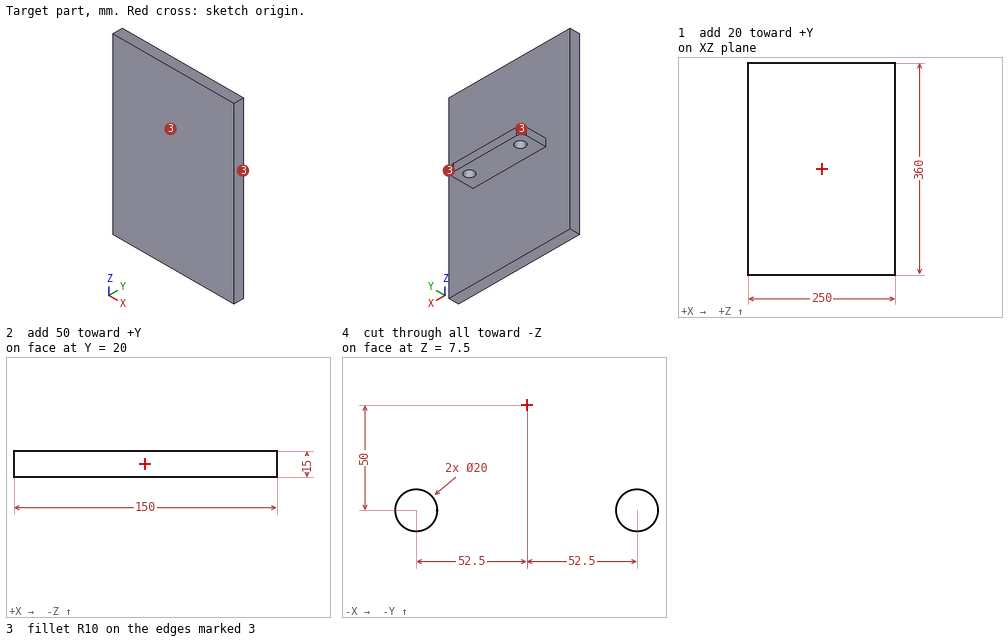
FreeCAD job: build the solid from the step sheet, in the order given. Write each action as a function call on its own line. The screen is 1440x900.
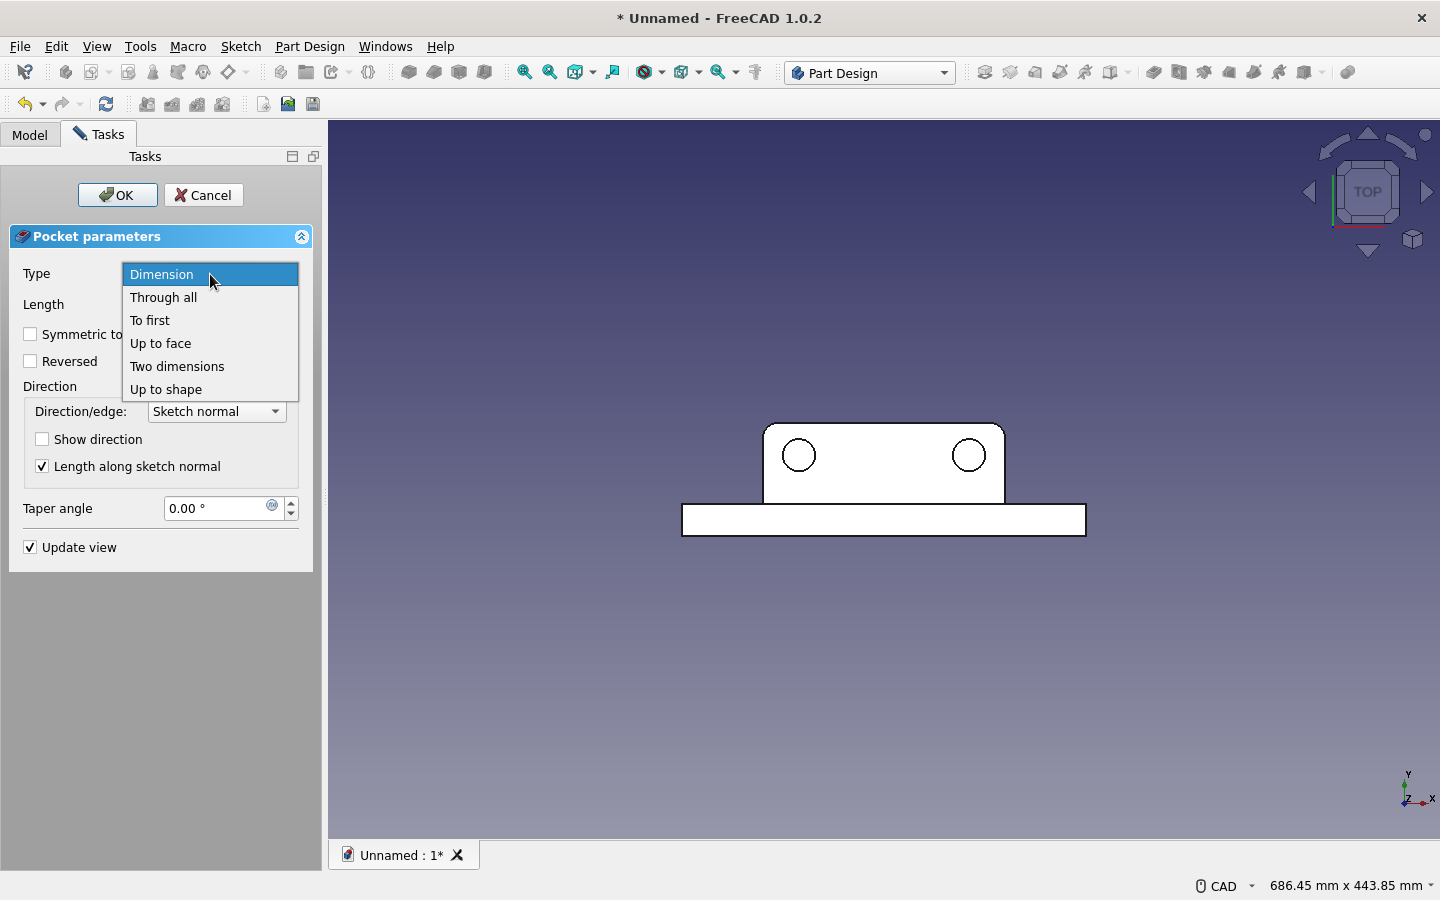
click(208, 298)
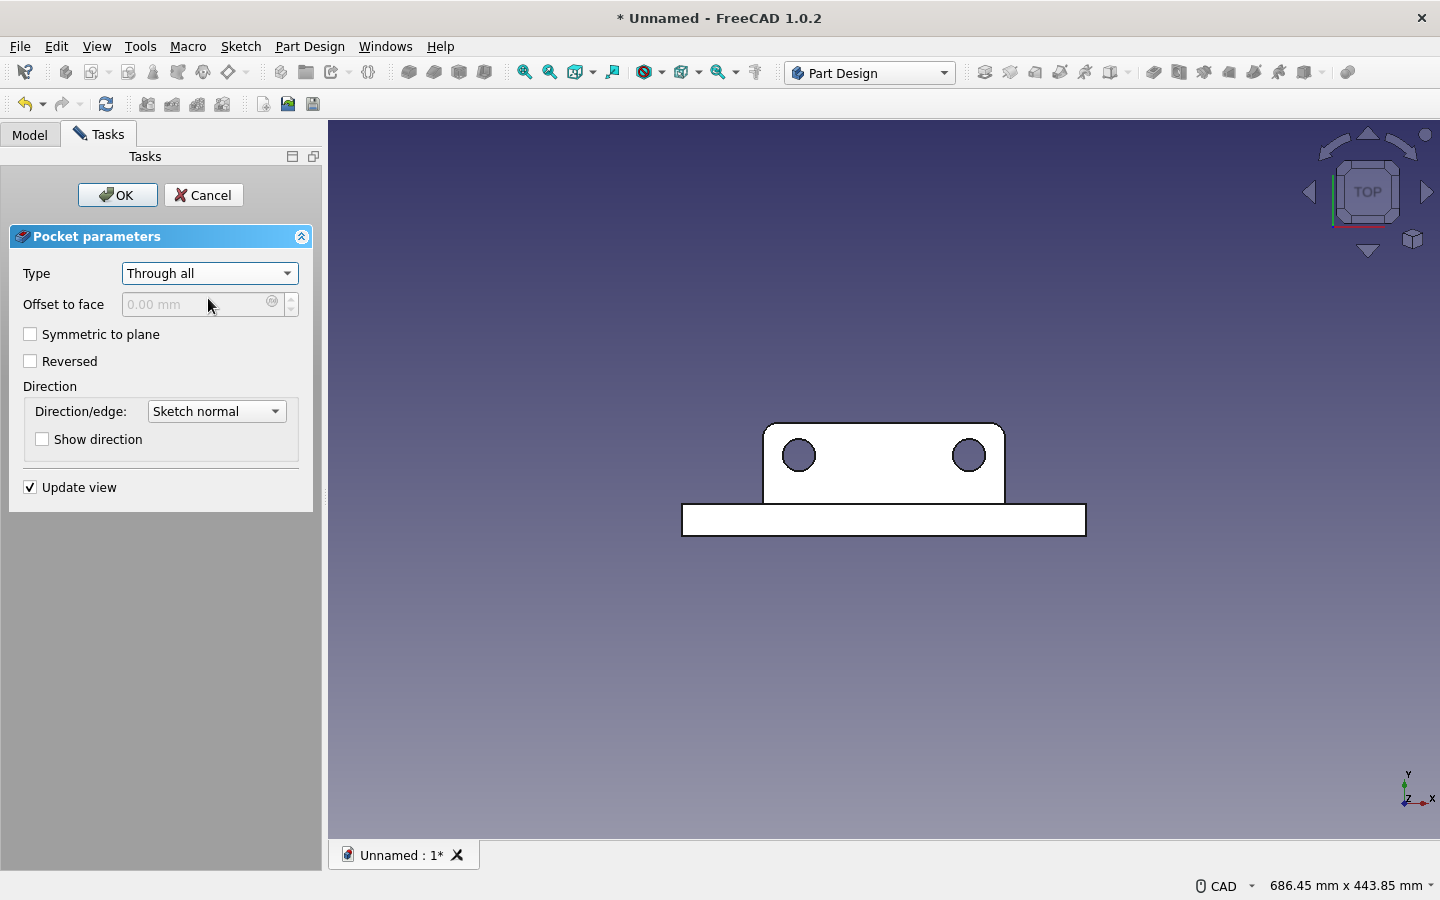
click(118, 195)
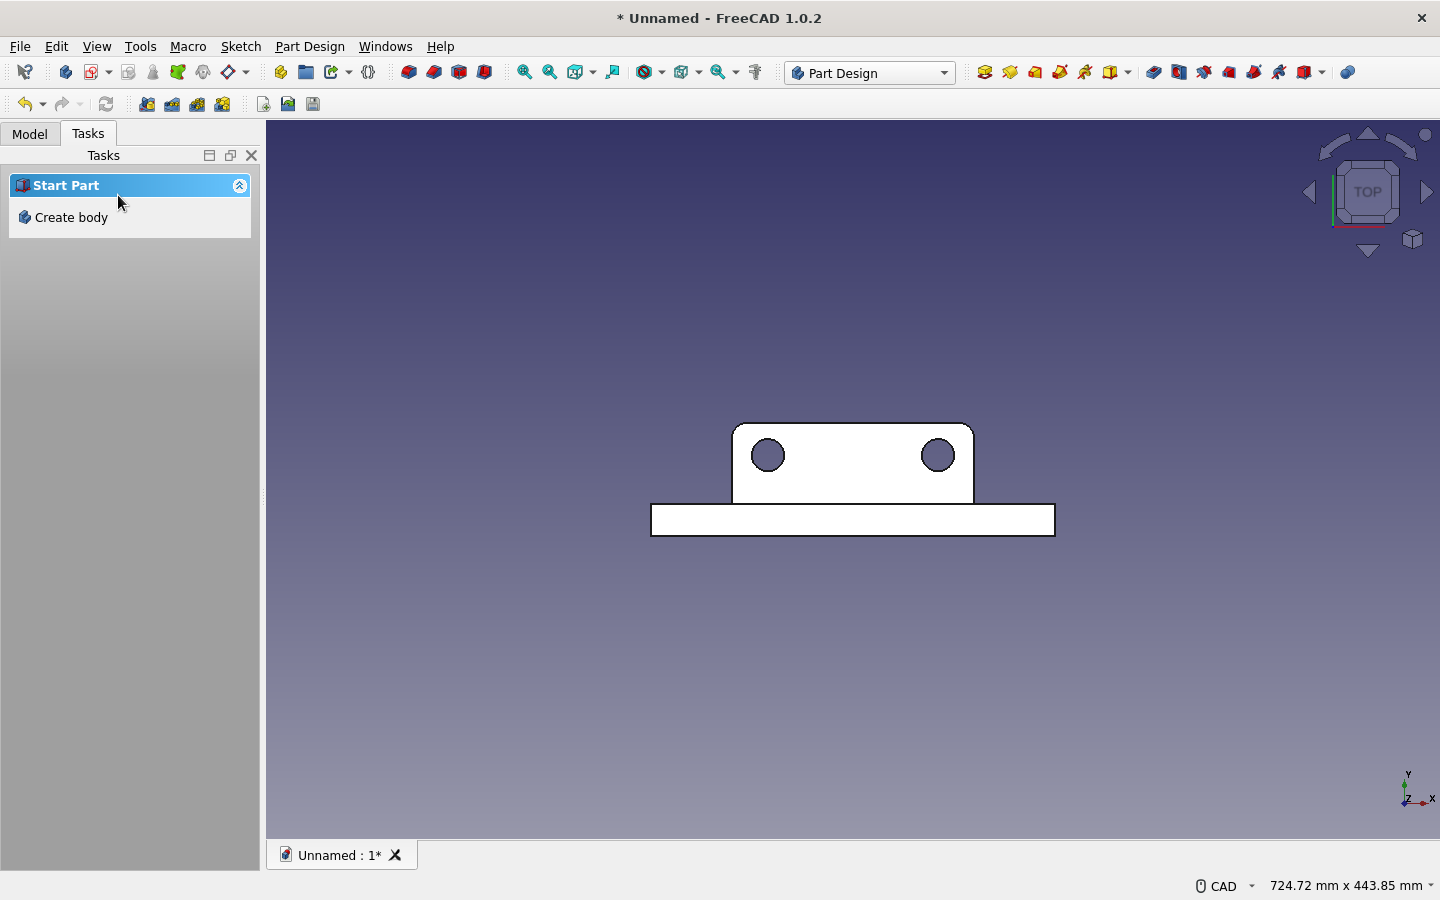
key(0)